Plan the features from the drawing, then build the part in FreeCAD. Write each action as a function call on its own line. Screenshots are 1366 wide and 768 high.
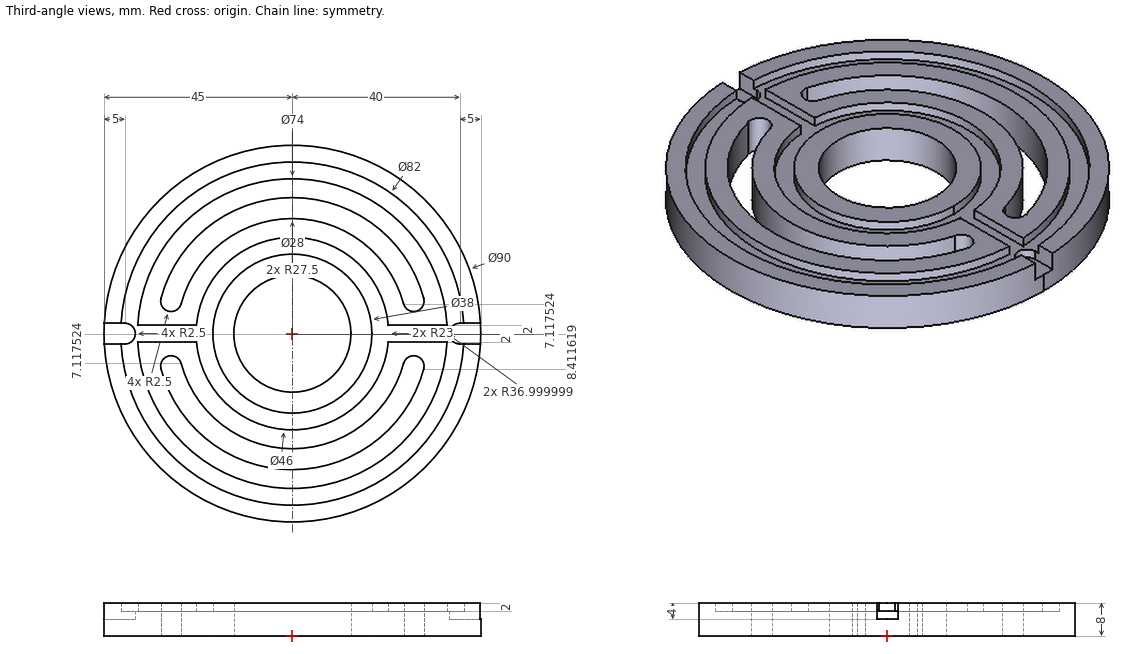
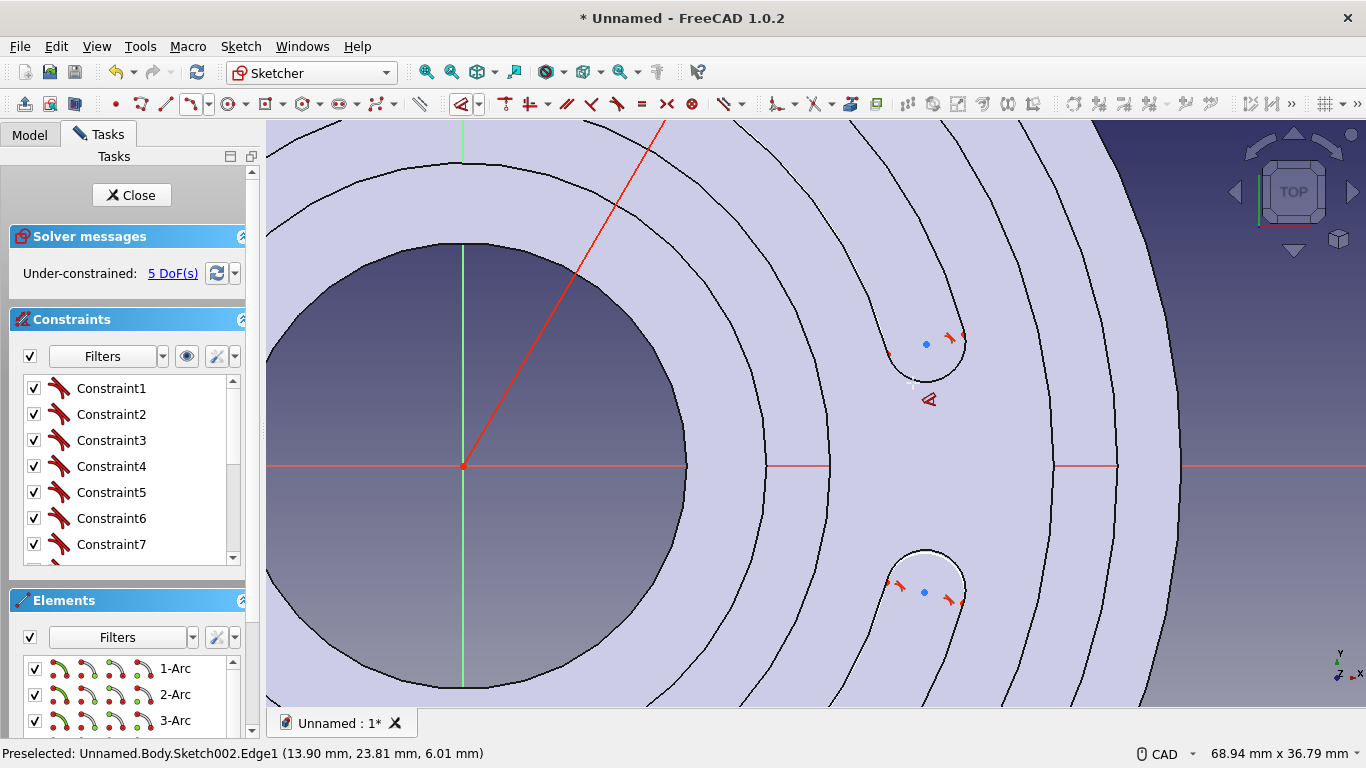
click(912, 381)
click(900, 411)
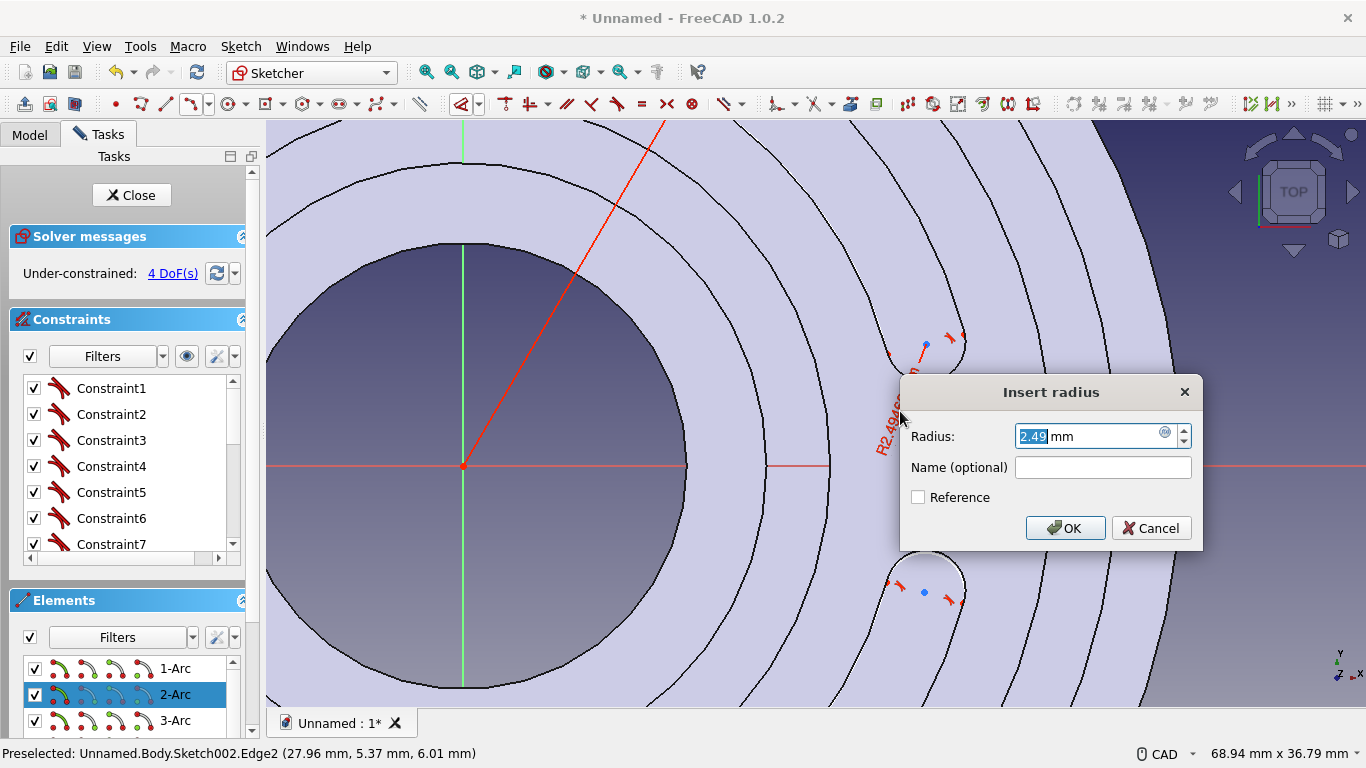
text(2.5)
key(Return)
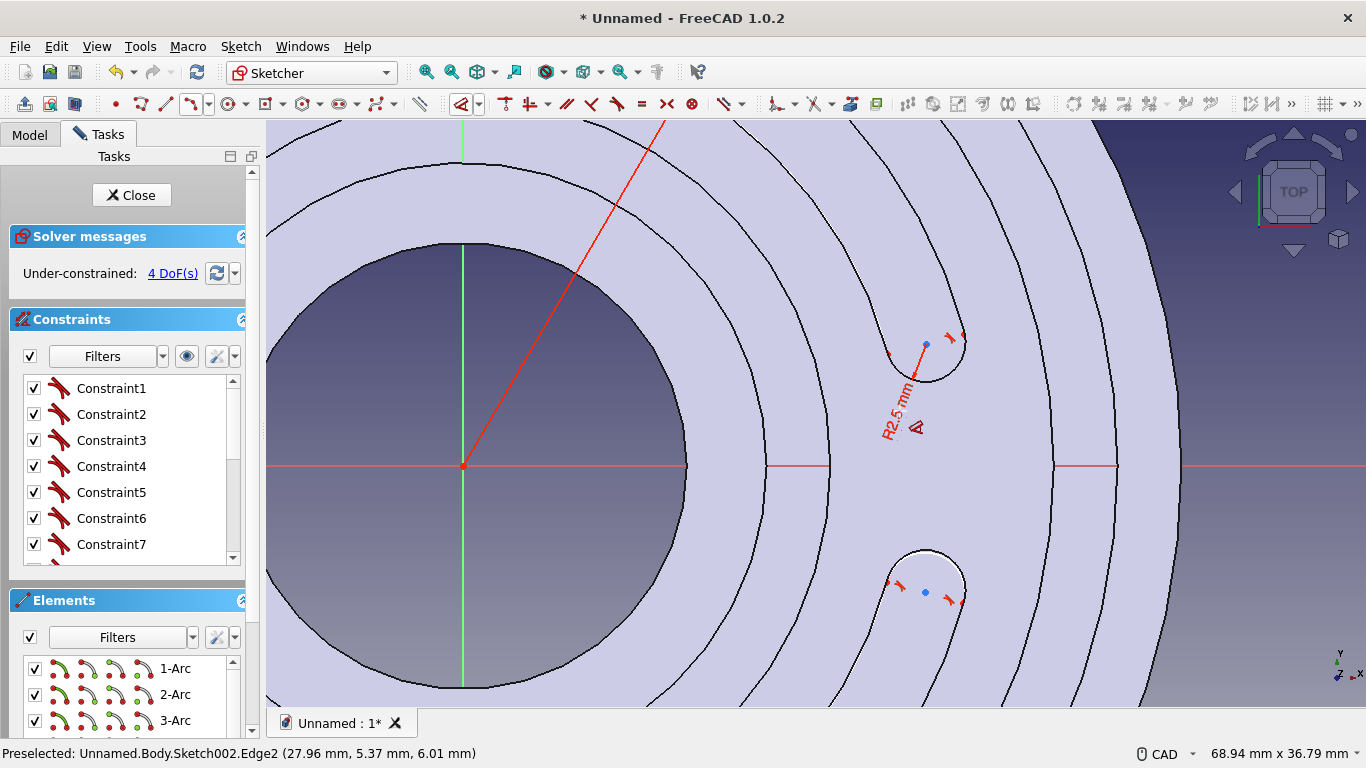
click(888, 354)
click(922, 436)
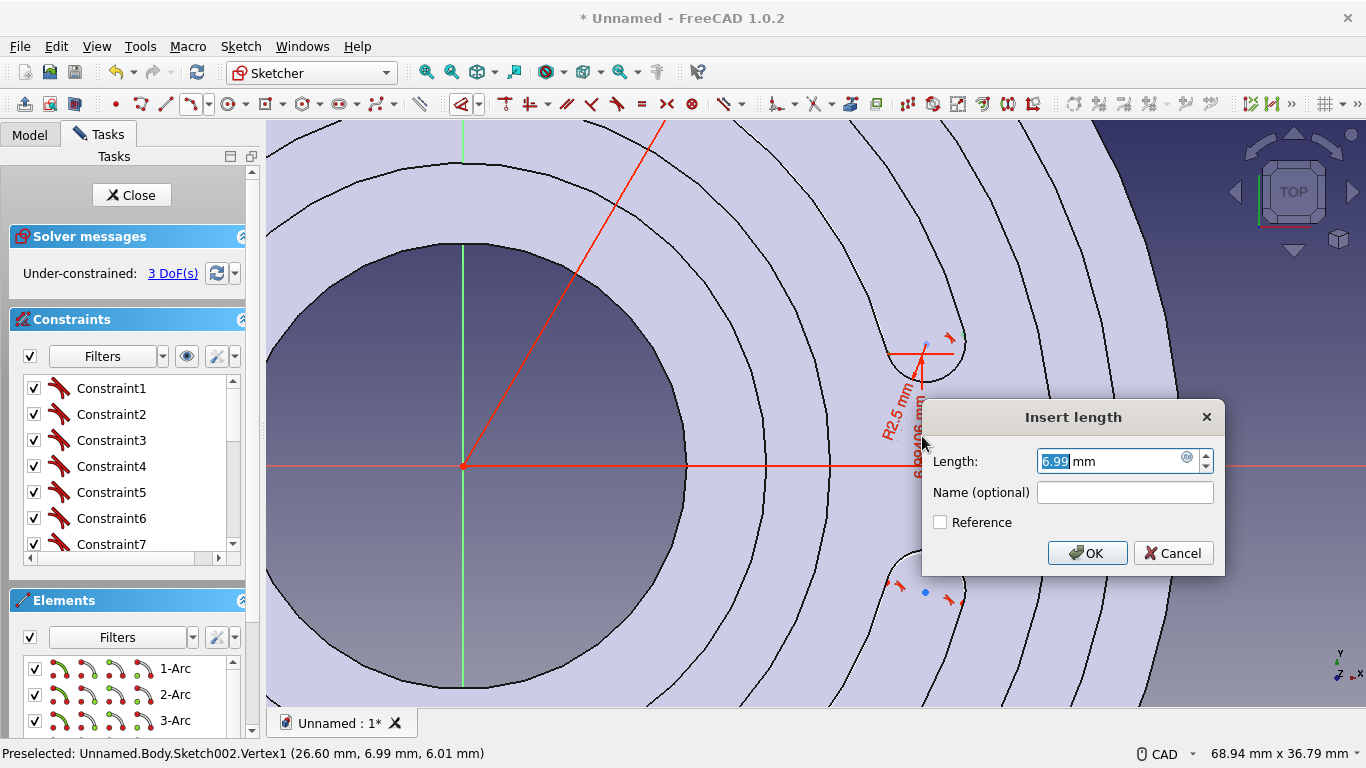
text(7.117524)
key(Return)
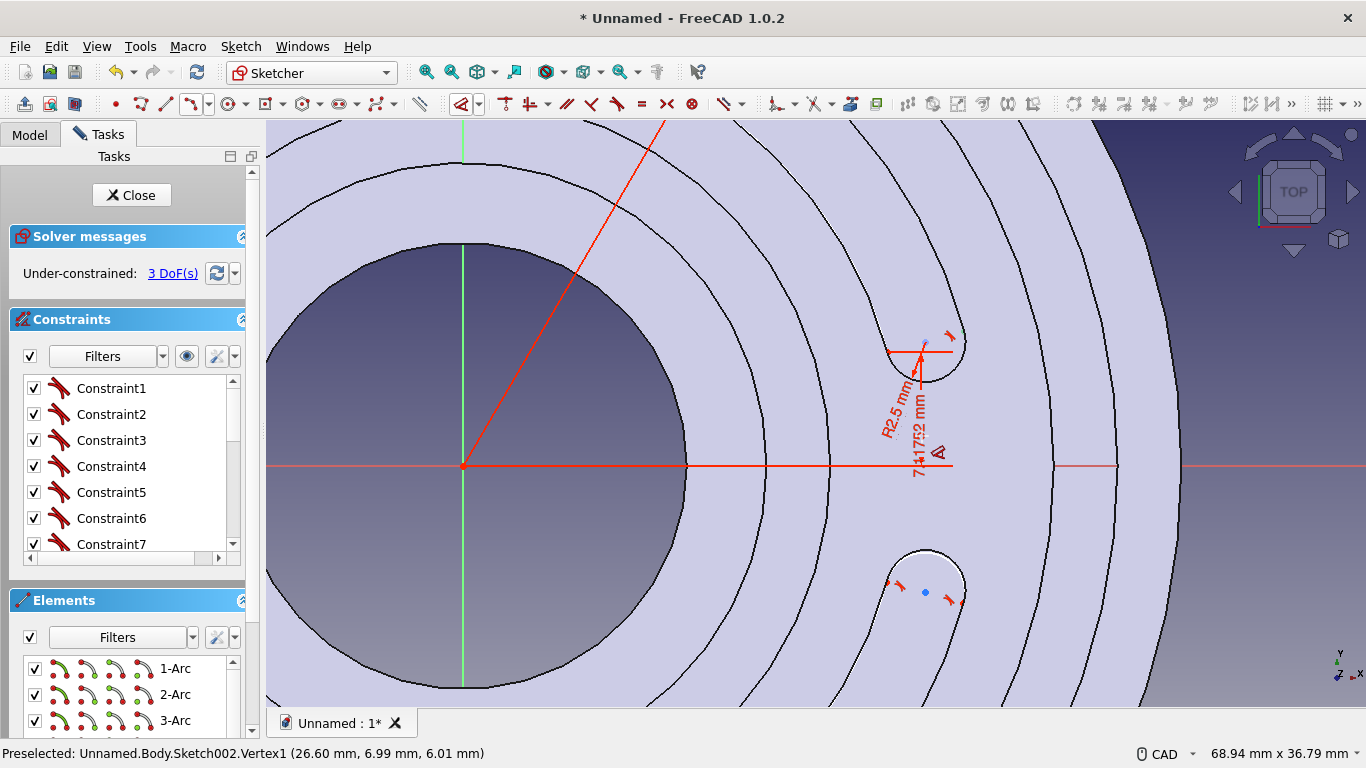
scroll(913, 383, down, 5)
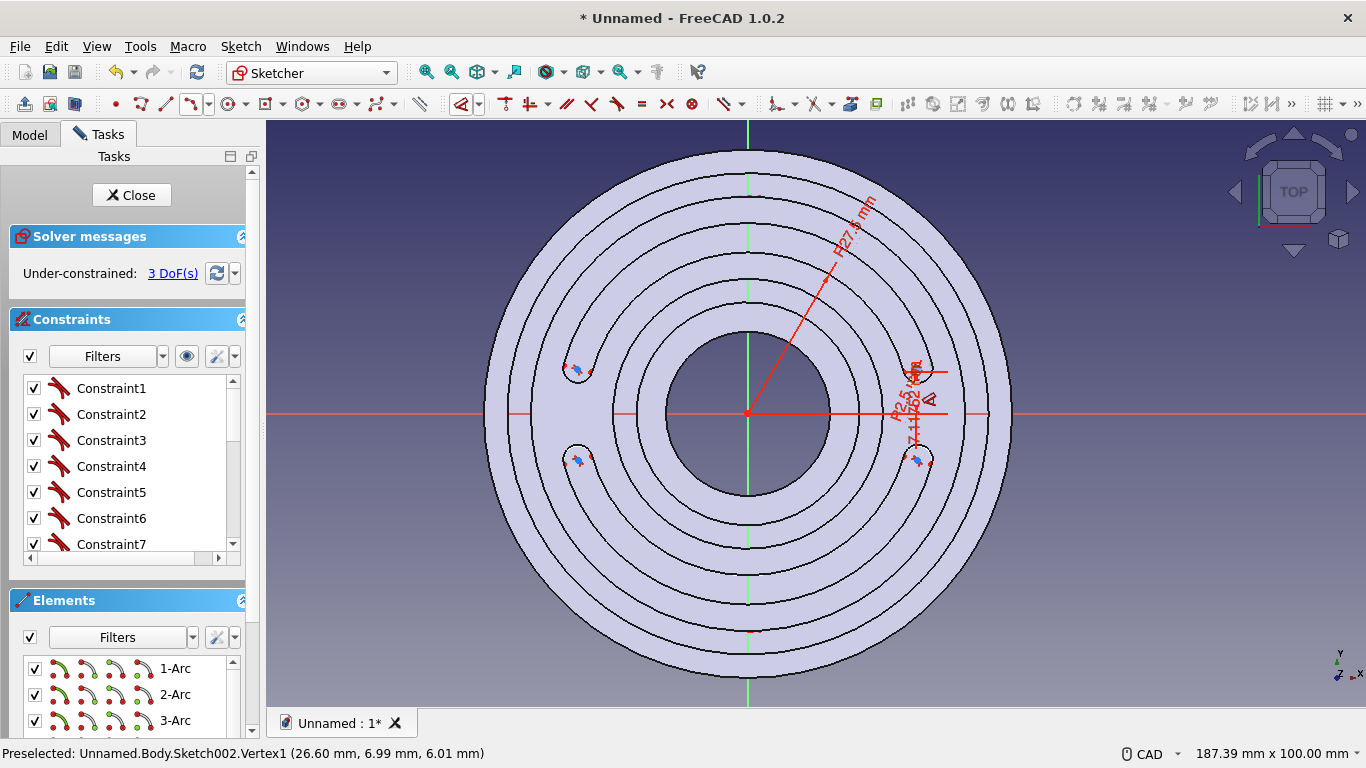
click(592, 373)
click(558, 393)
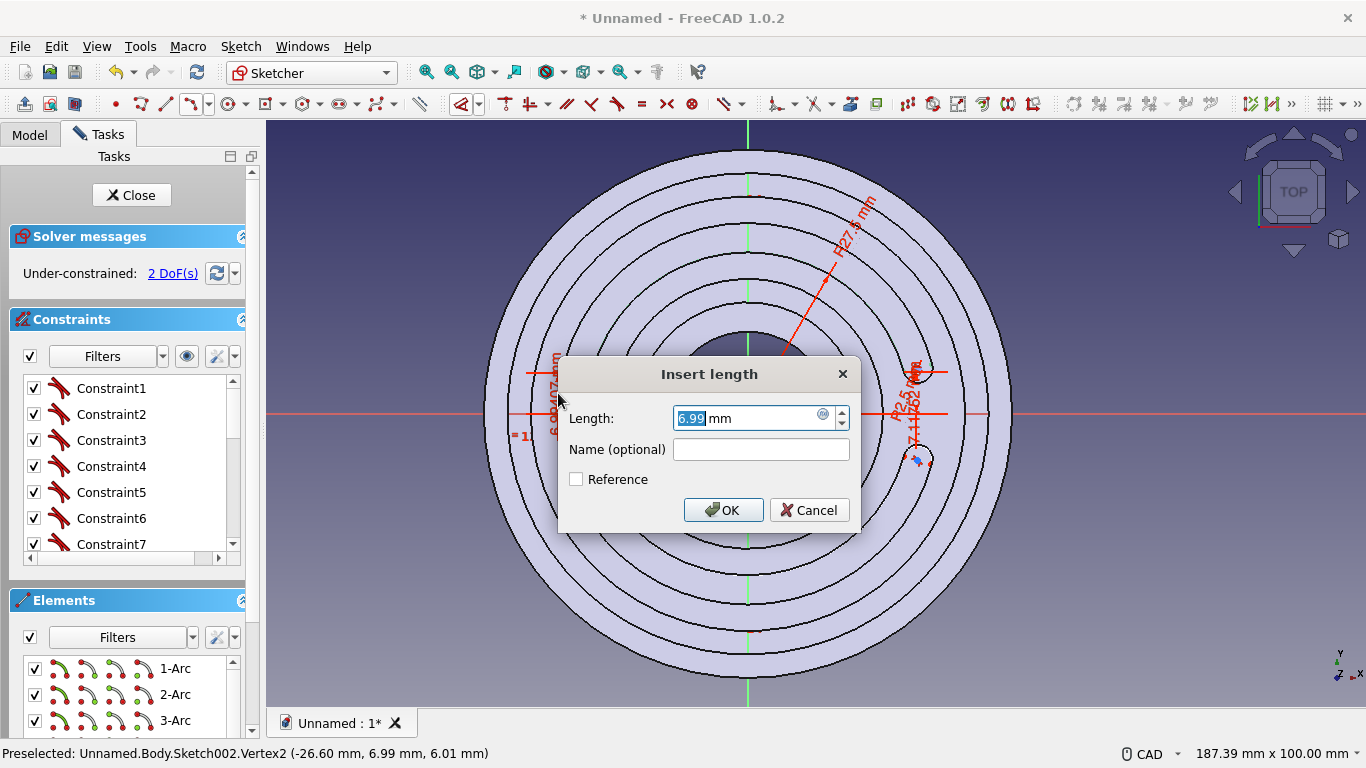
text(7.117524)
key(Return)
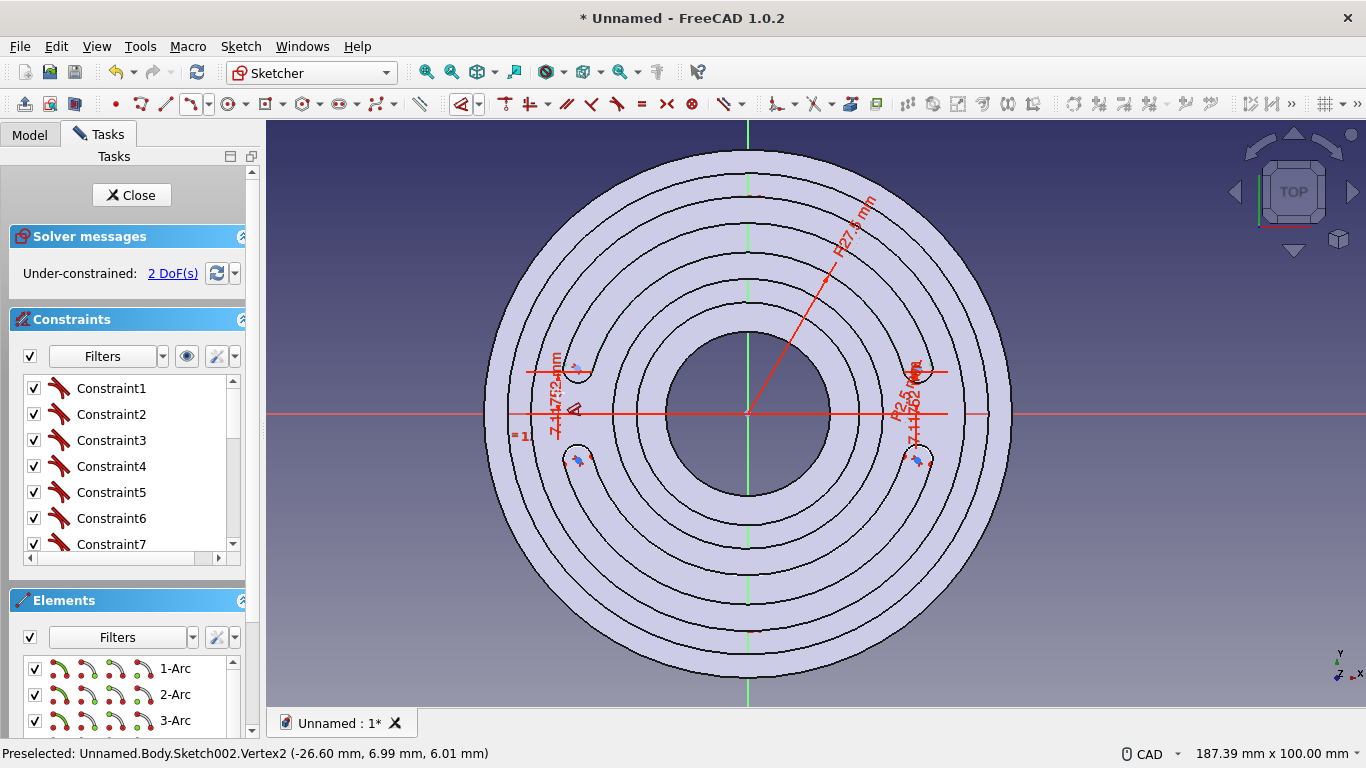
click(592, 457)
click(558, 435)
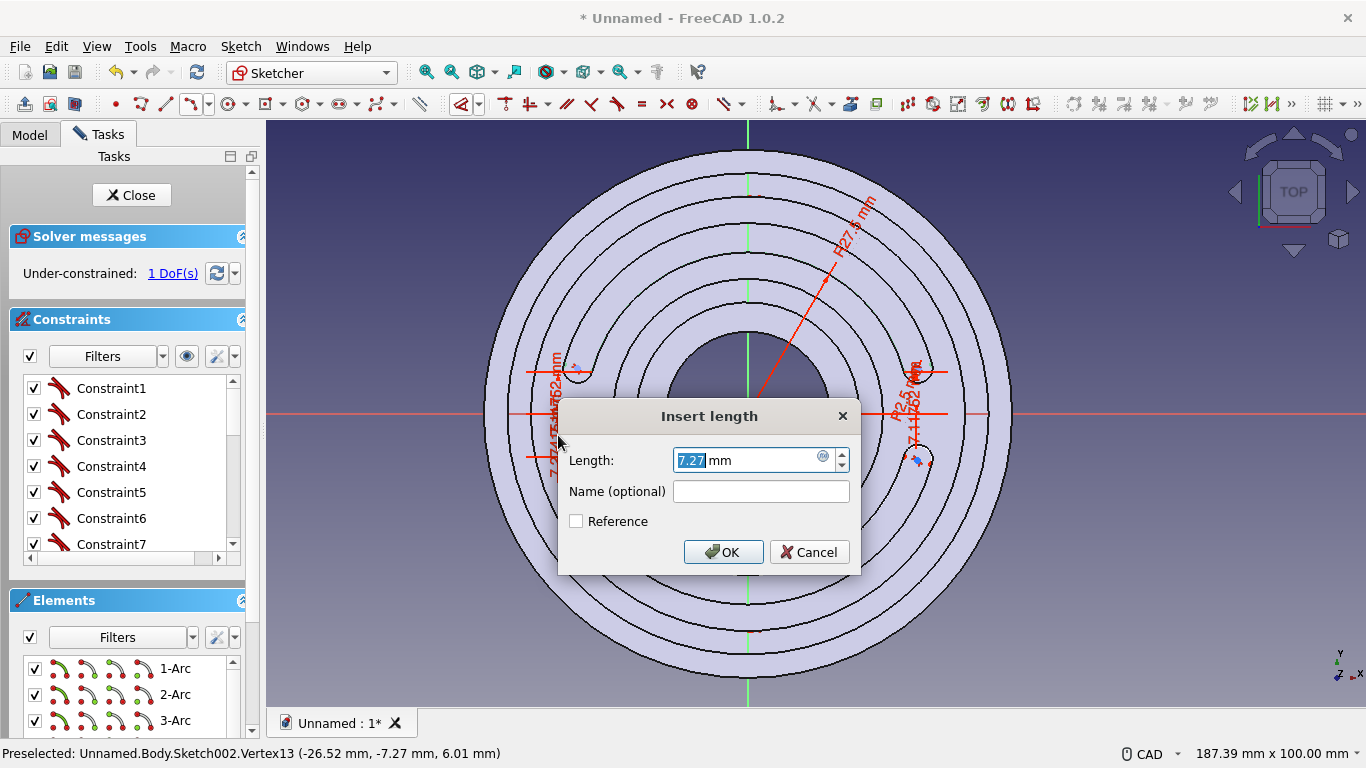
text(7.117524)
key(Return)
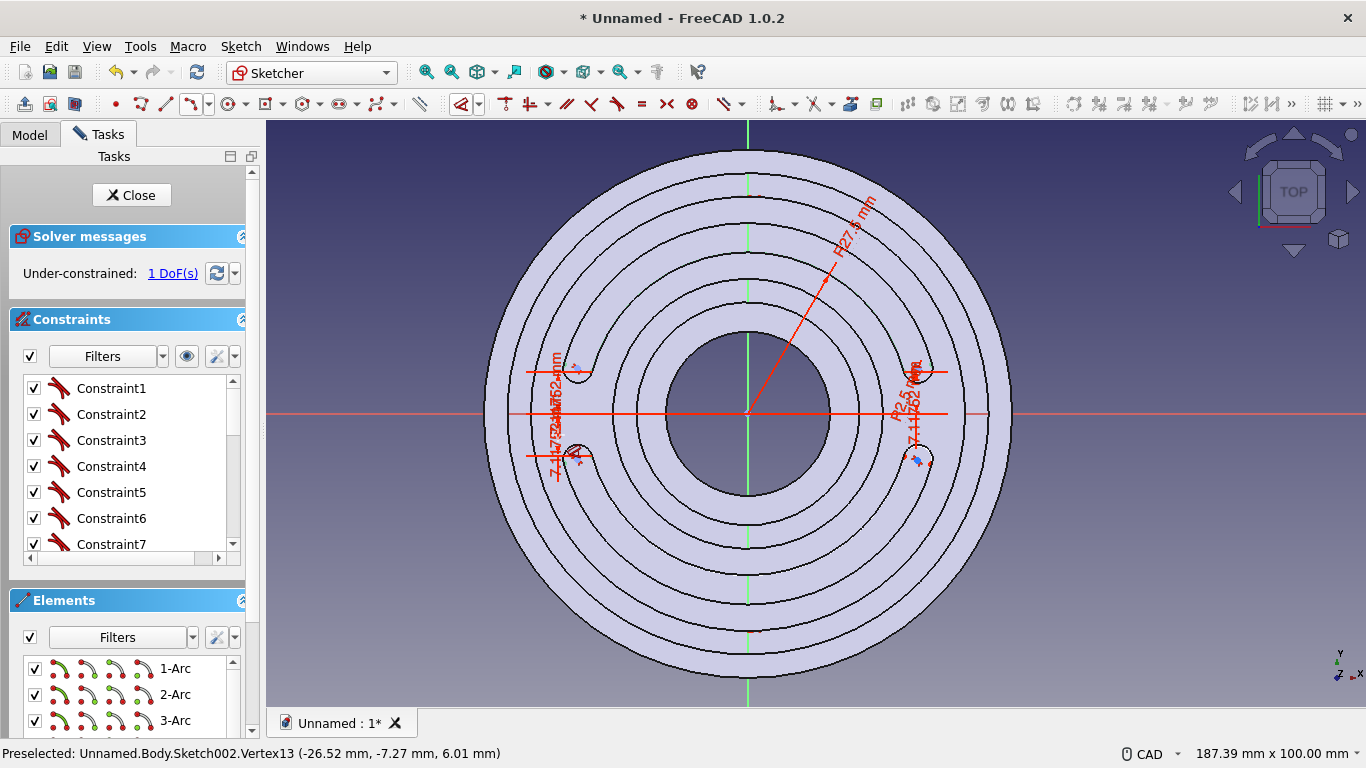
click(932, 464)
click(966, 439)